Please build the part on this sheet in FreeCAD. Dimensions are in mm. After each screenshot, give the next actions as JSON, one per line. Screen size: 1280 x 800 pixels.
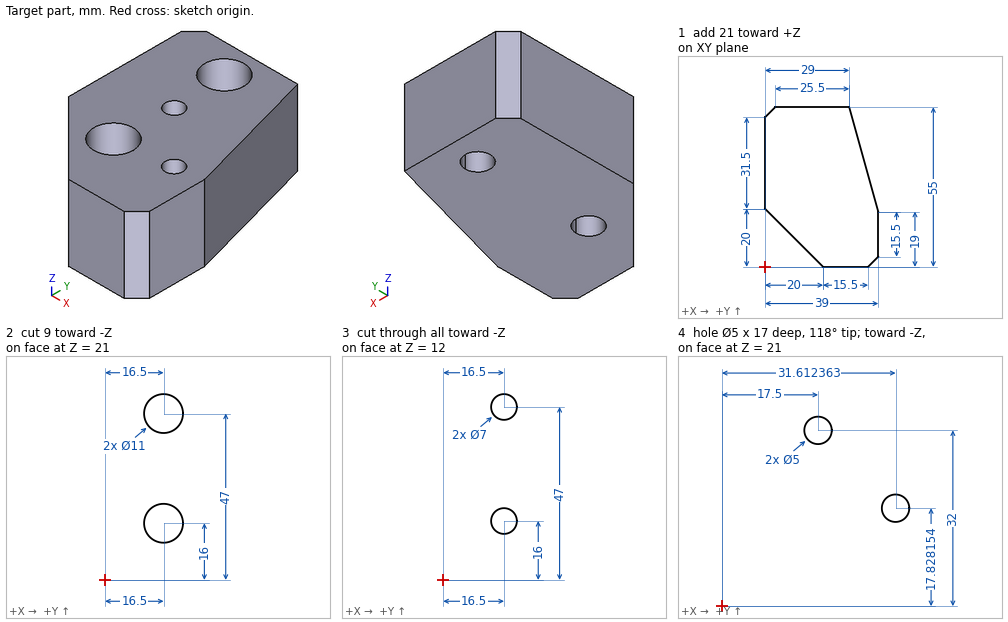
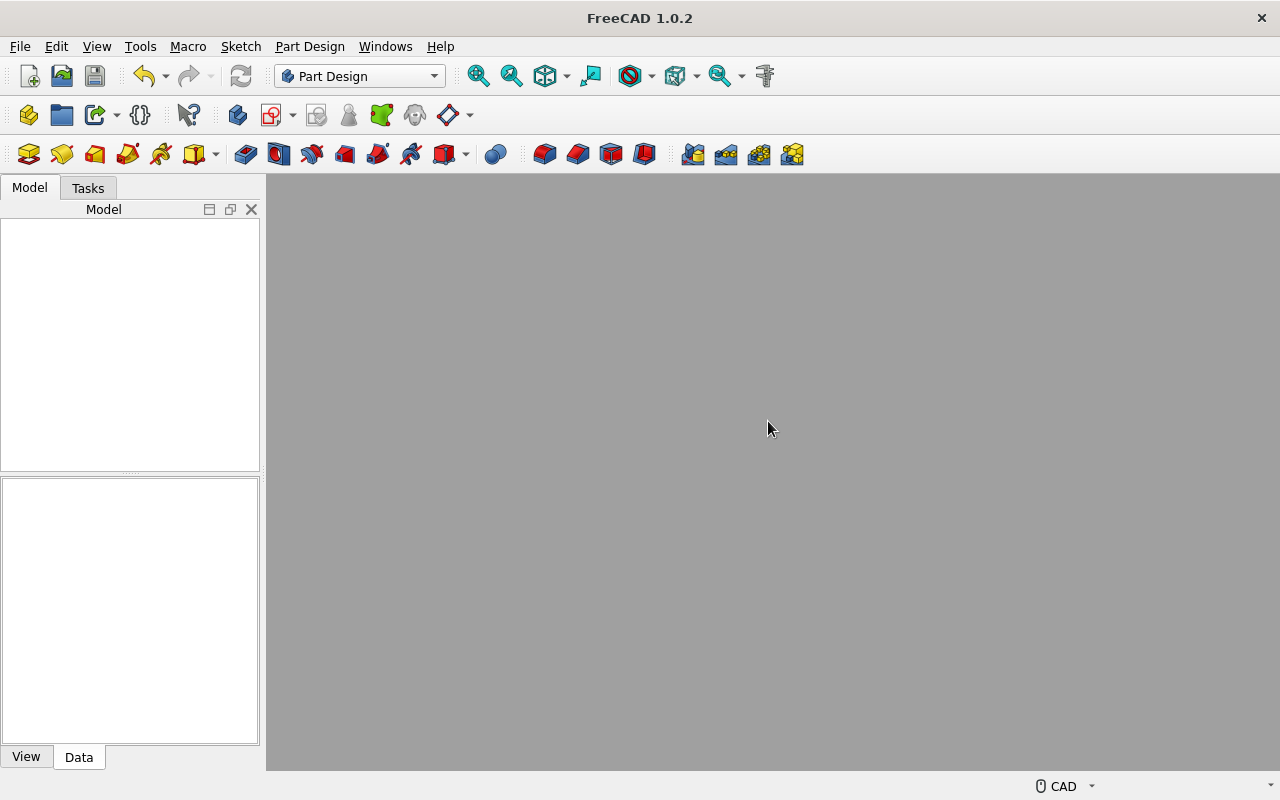
{"action": "left_click", "coordinate": [29, 76]}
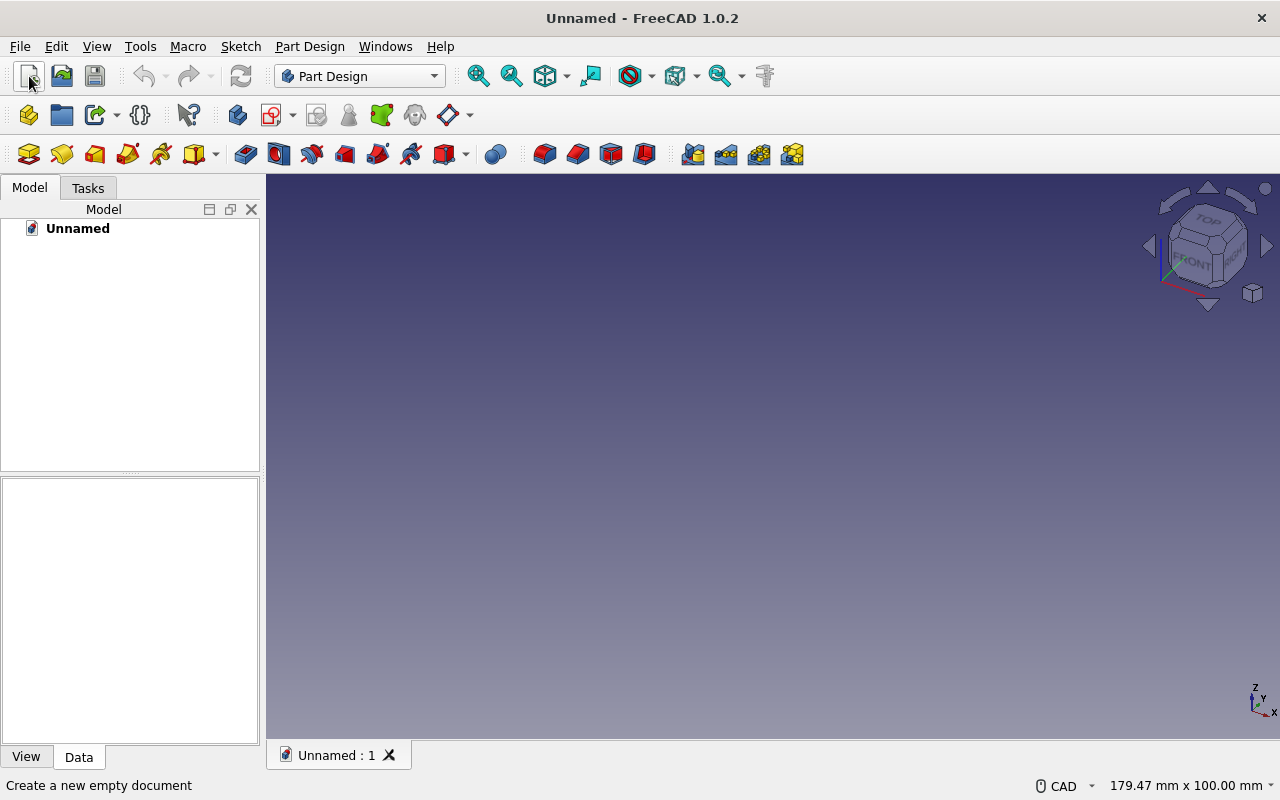
{"action": "left_click", "coordinate": [270, 116]}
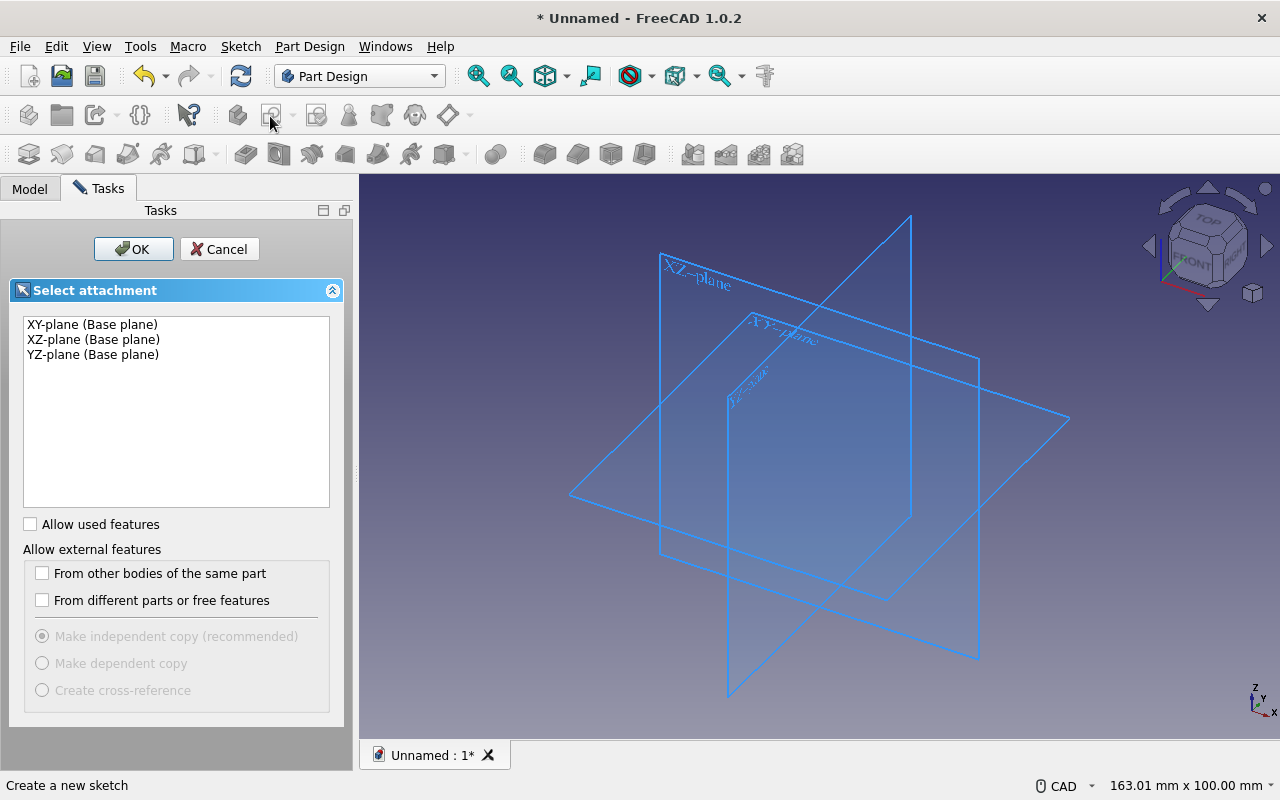
{"action": "left_click", "coordinate": [84, 324]}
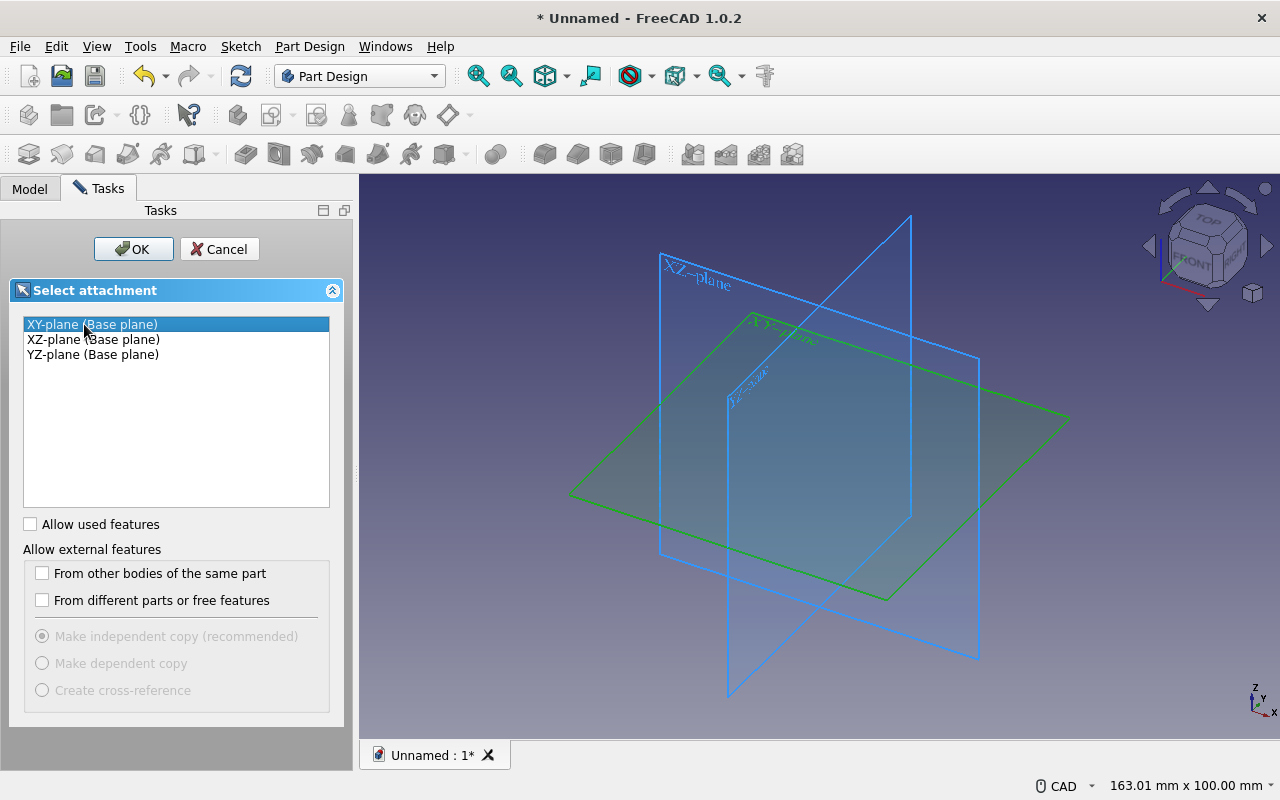
{"action": "left_click", "coordinate": [134, 249]}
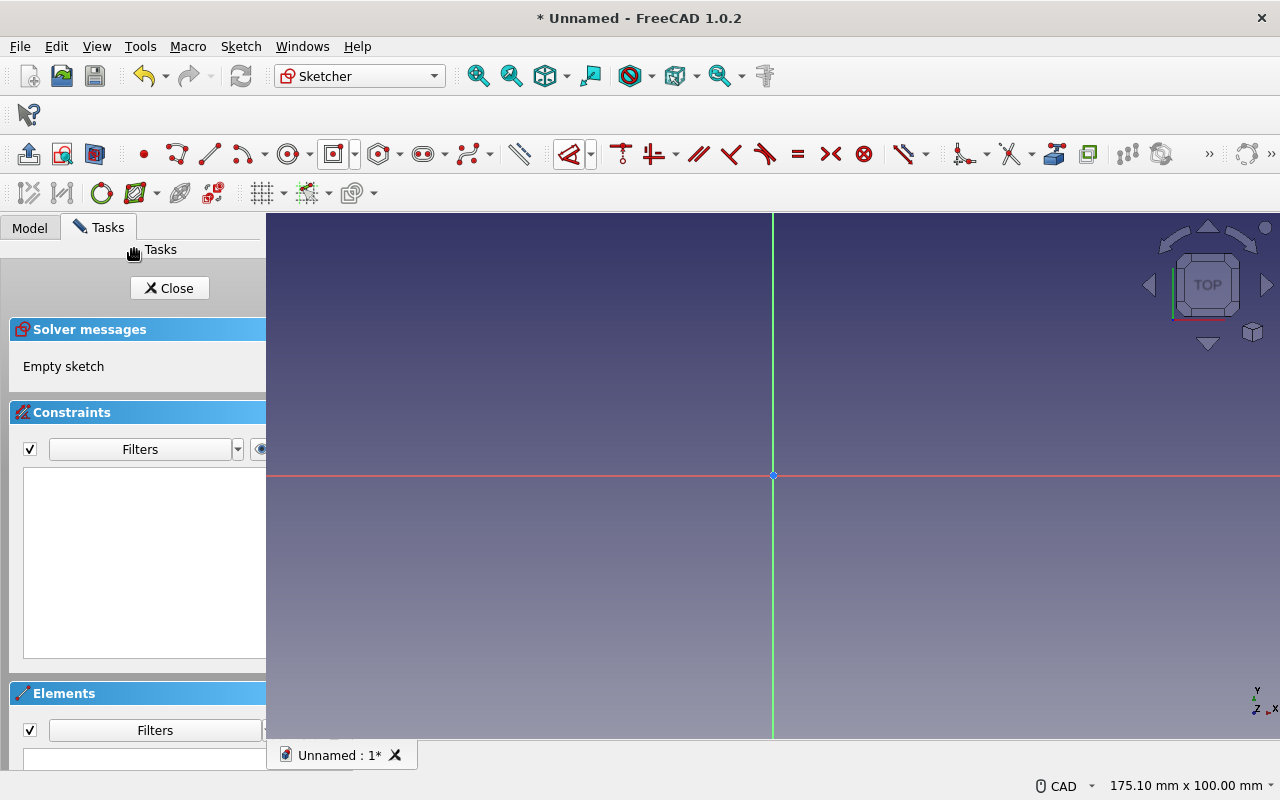
{"action": "scroll", "coordinate": [294, 711], "scroll_direction": "down", "scroll_amount": 1}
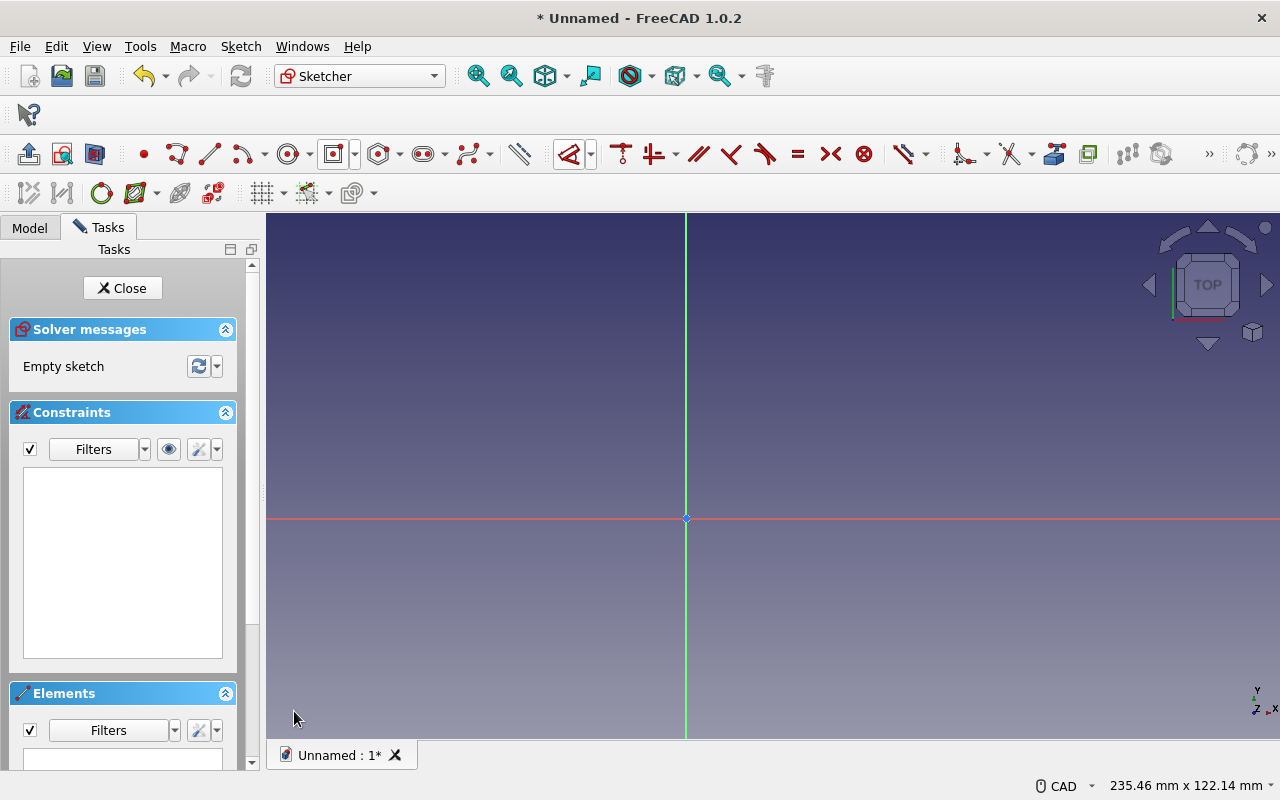
{"action": "scroll", "coordinate": [904, 247], "scroll_direction": "up", "scroll_amount": 2}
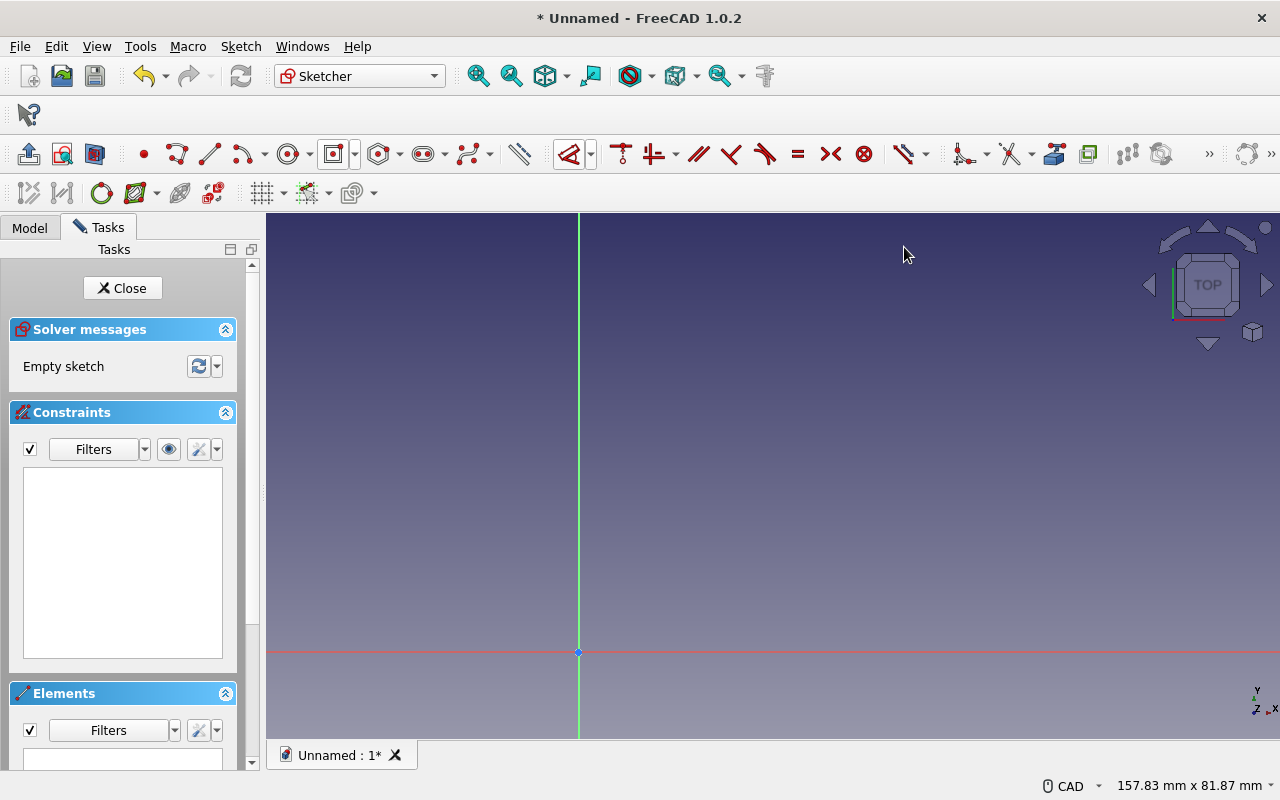
{"action": "left_click", "coordinate": [177, 154]}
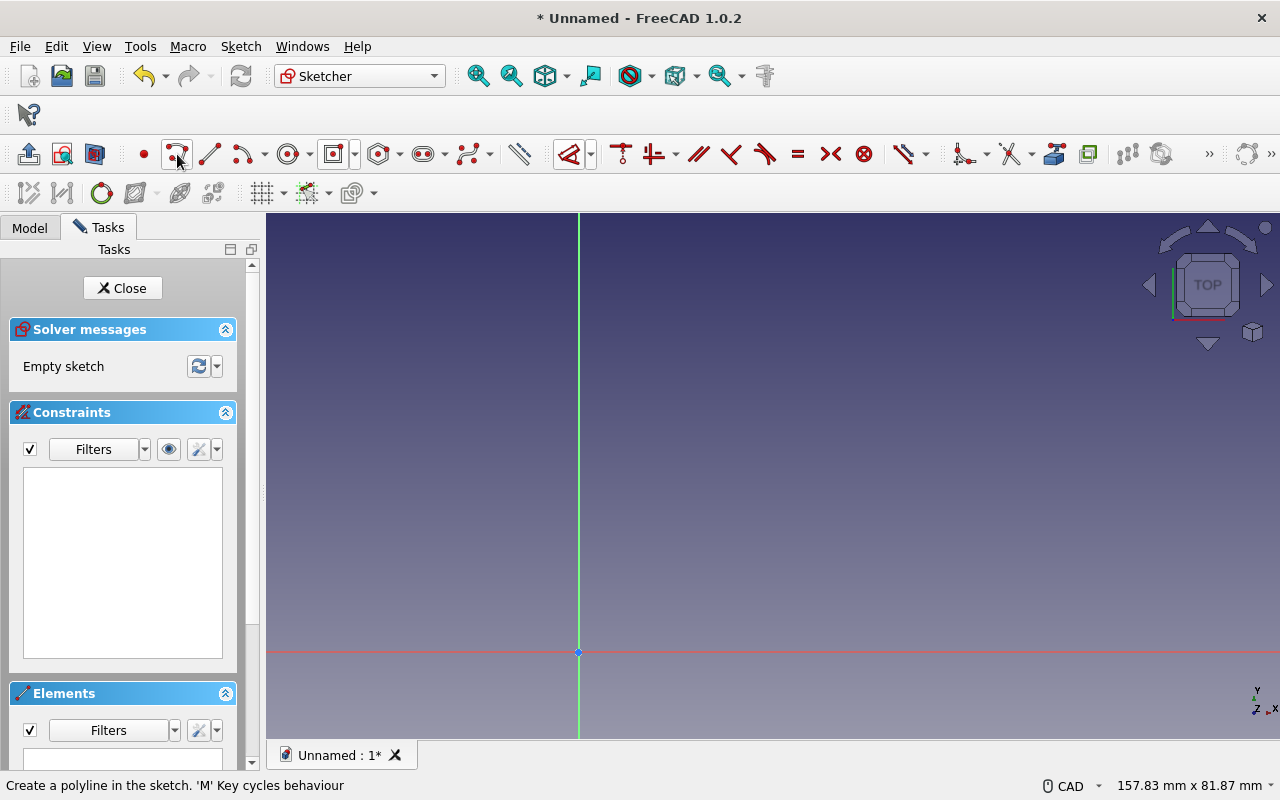
{"action": "left_click", "coordinate": [579, 524]}
{"action": "left_click", "coordinate": [707, 652]}
{"action": "left_click", "coordinate": [807, 643]}
{"action": "left_click", "coordinate": [829, 630]}
{"action": "left_click", "coordinate": [829, 530]}
{"action": "left_click", "coordinate": [765, 299]}
{"action": "left_click", "coordinate": [601, 299]}
{"action": "left_click", "coordinate": [588, 322]}
{"action": "left_click", "coordinate": [579, 525]}
{"action": "key", "text": "Escape"}
{"action": "key", "text": "Escape"}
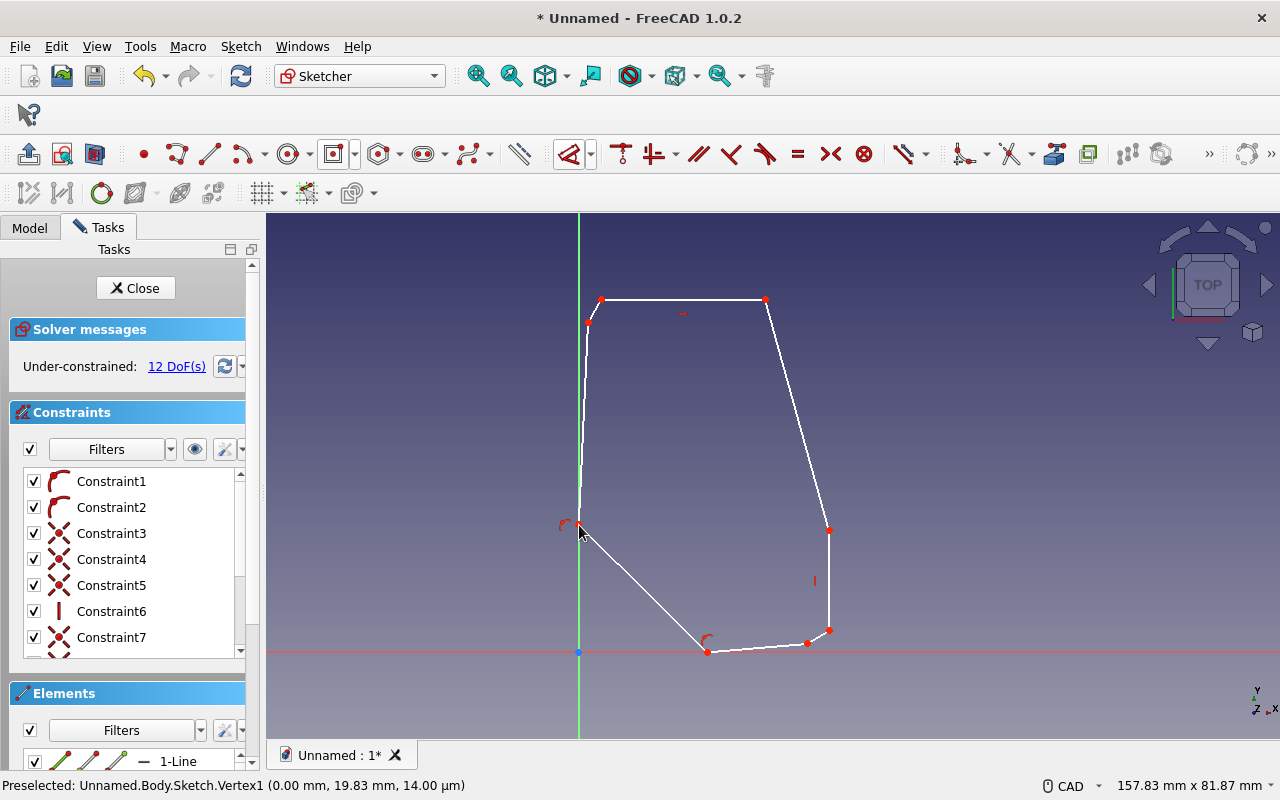
{"action": "left_click", "coordinate": [737, 650]}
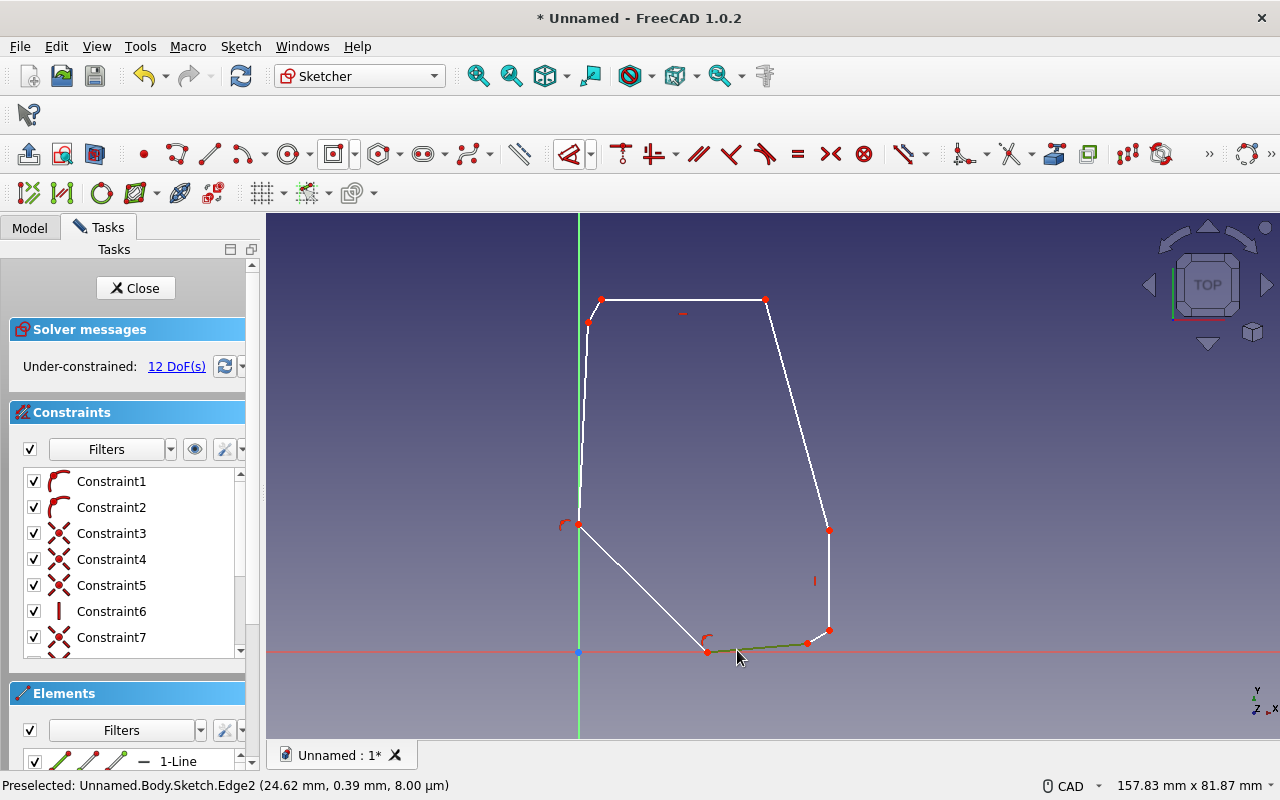
{"action": "left_click", "coordinate": [676, 154]}